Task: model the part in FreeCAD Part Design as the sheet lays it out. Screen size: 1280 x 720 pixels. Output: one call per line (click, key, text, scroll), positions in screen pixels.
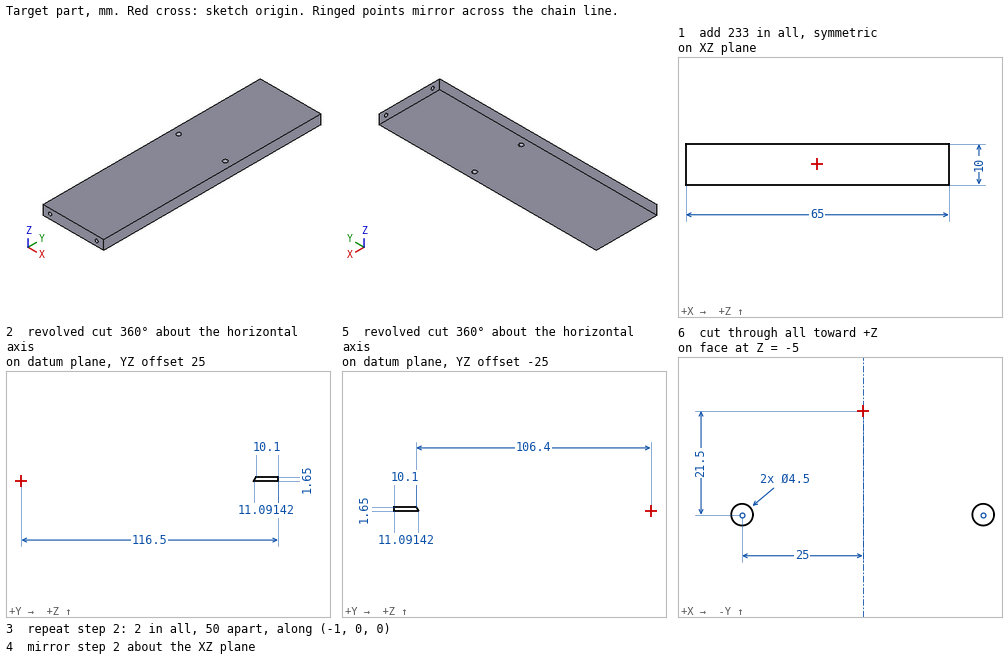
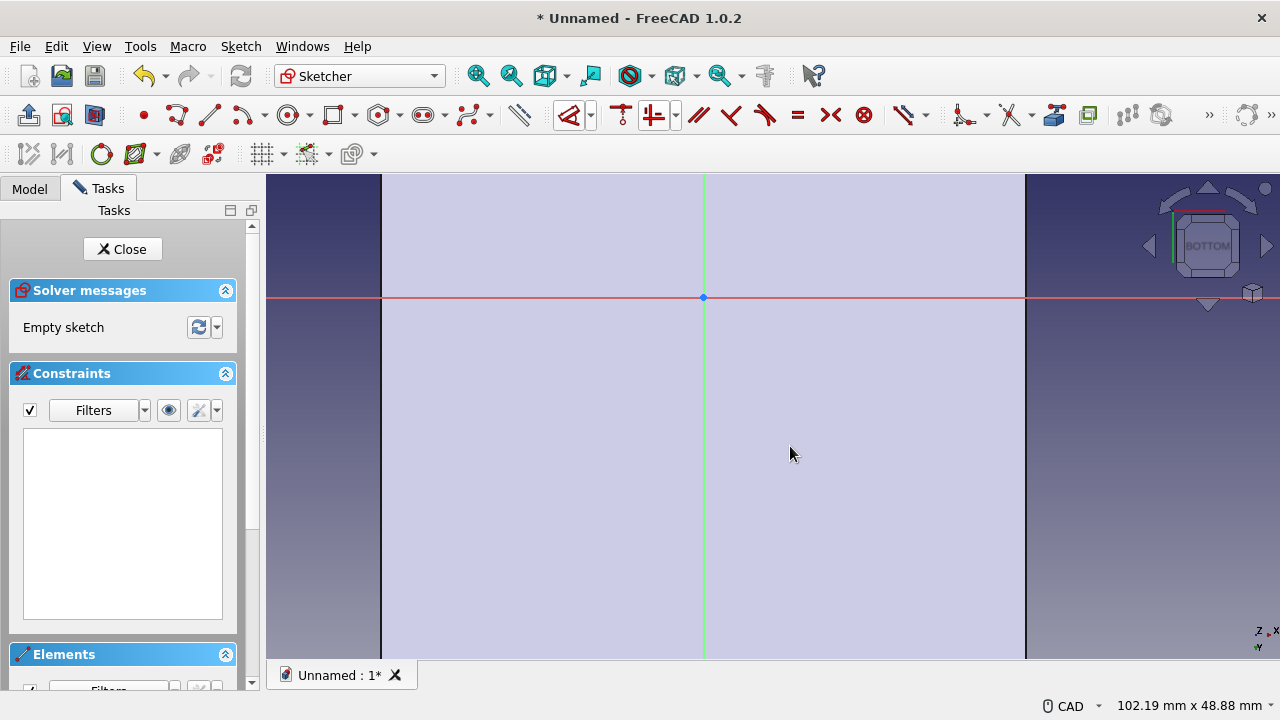
key(g)
key(c)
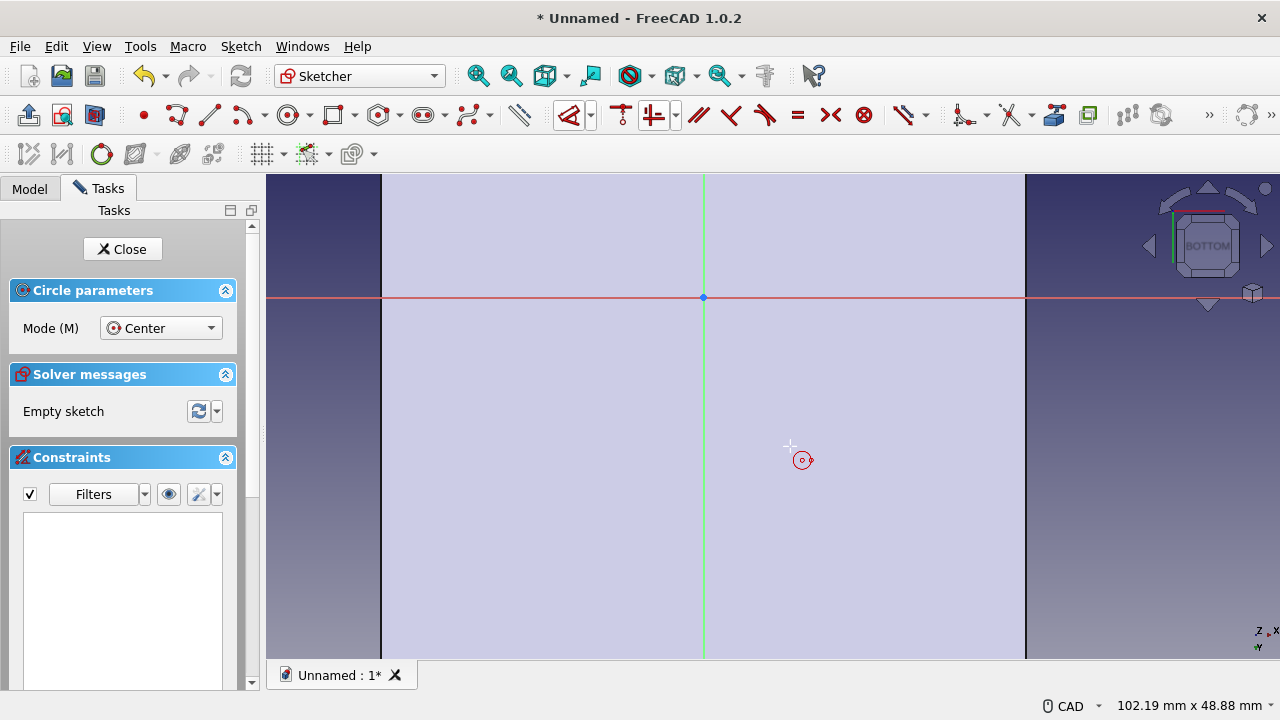
click(456, 511)
click(471, 495)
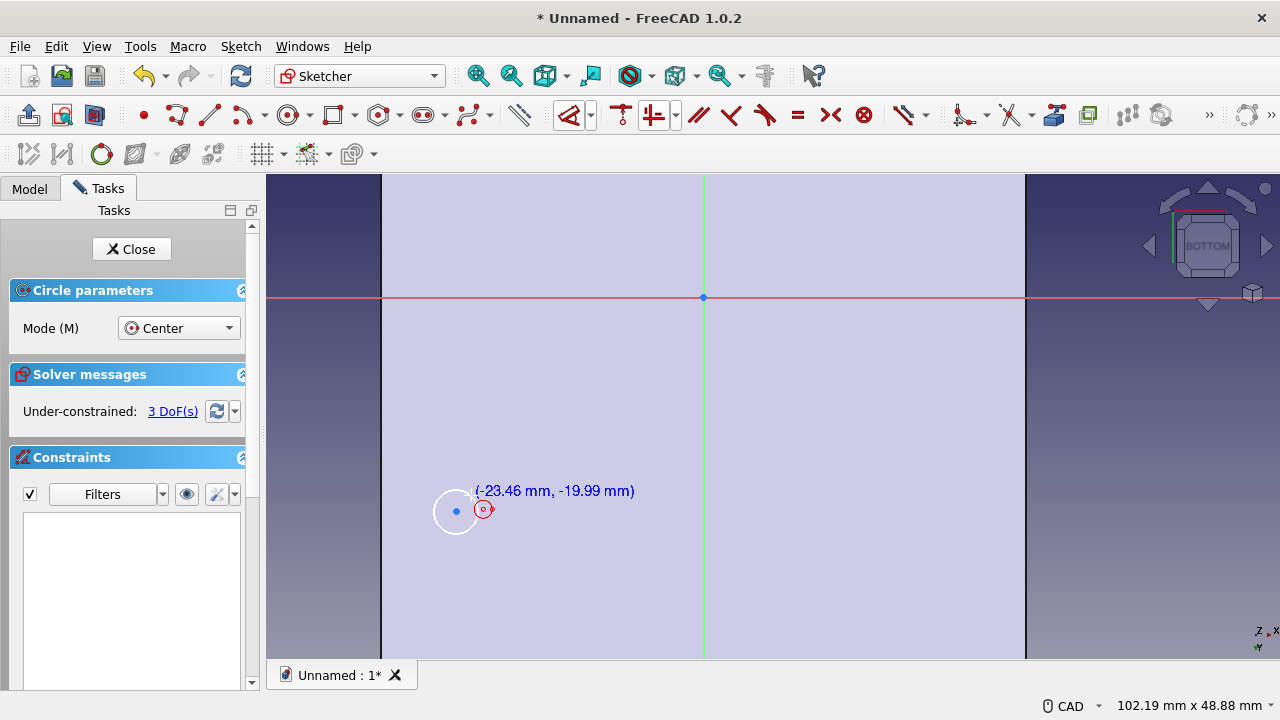
click(952, 511)
click(968, 495)
key(Escape)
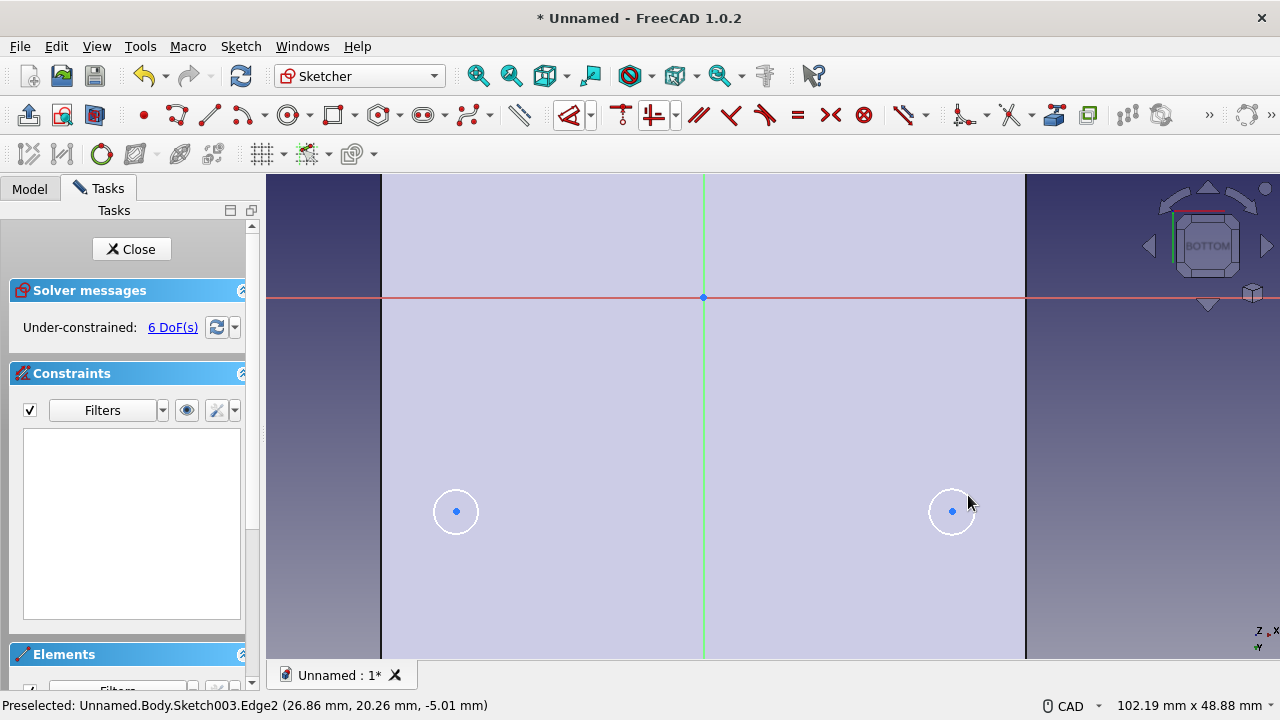
click(471, 496)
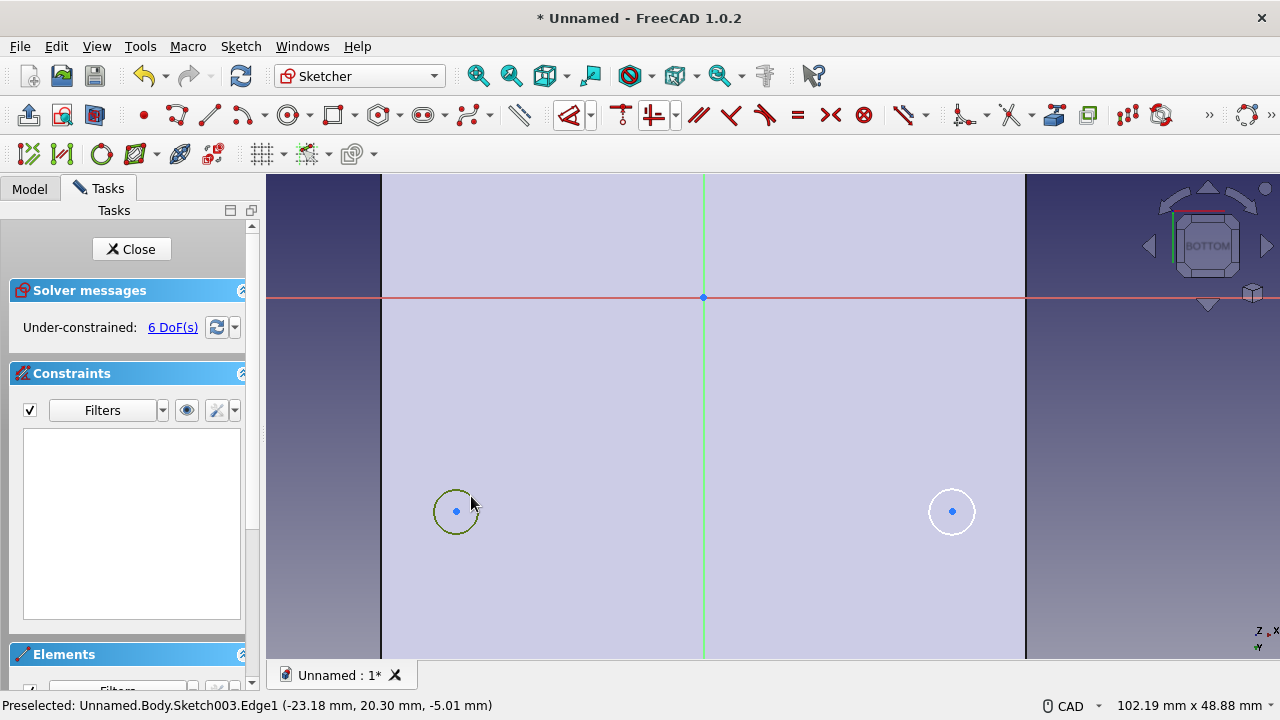
click(968, 496)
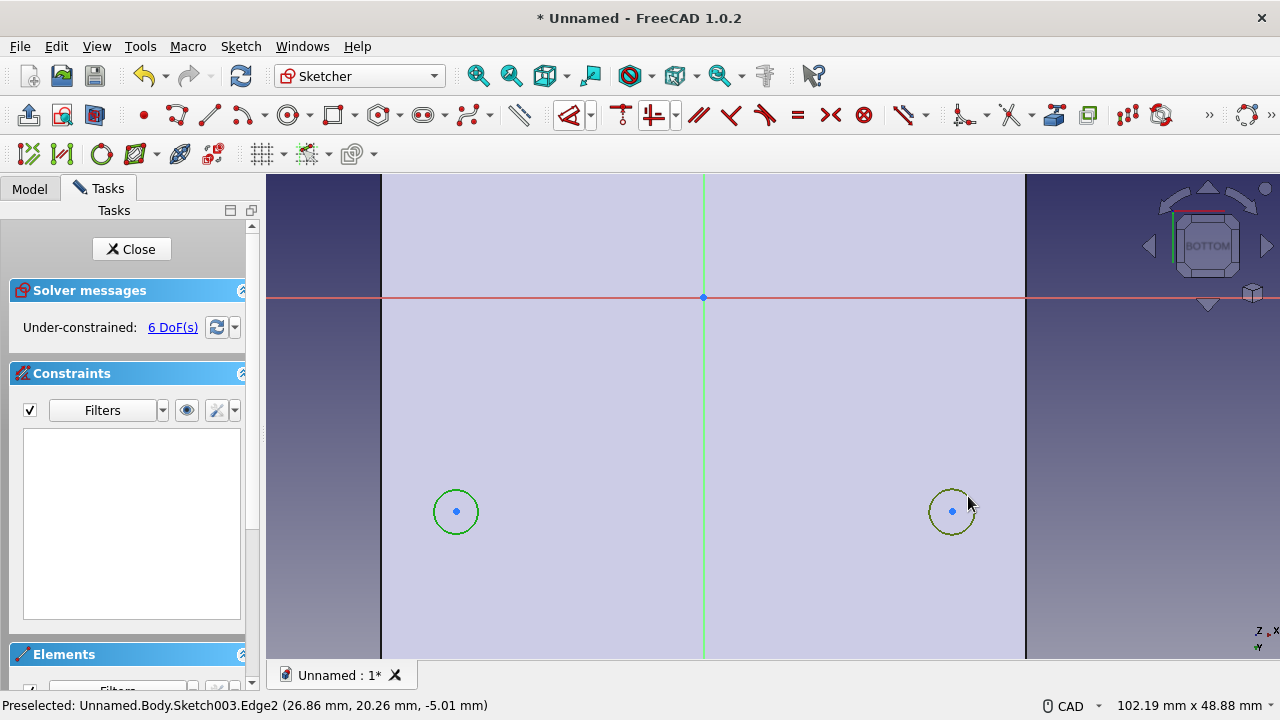
key(e)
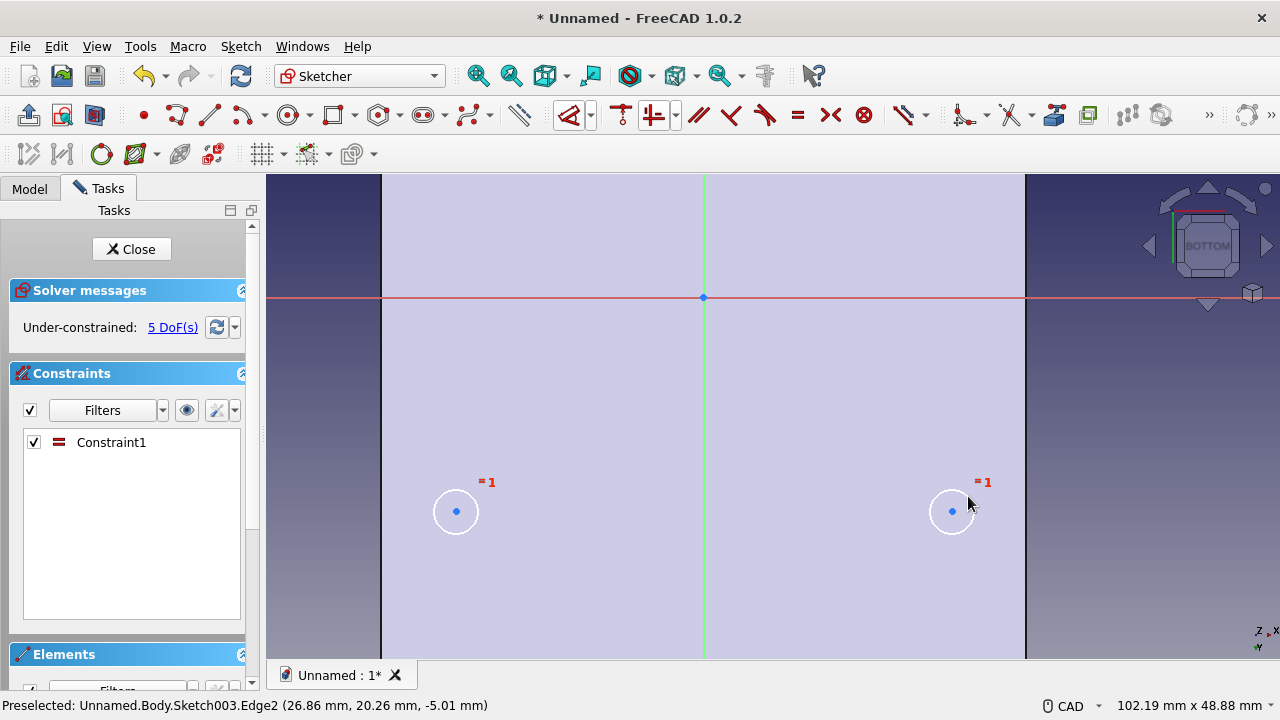
click(456, 512)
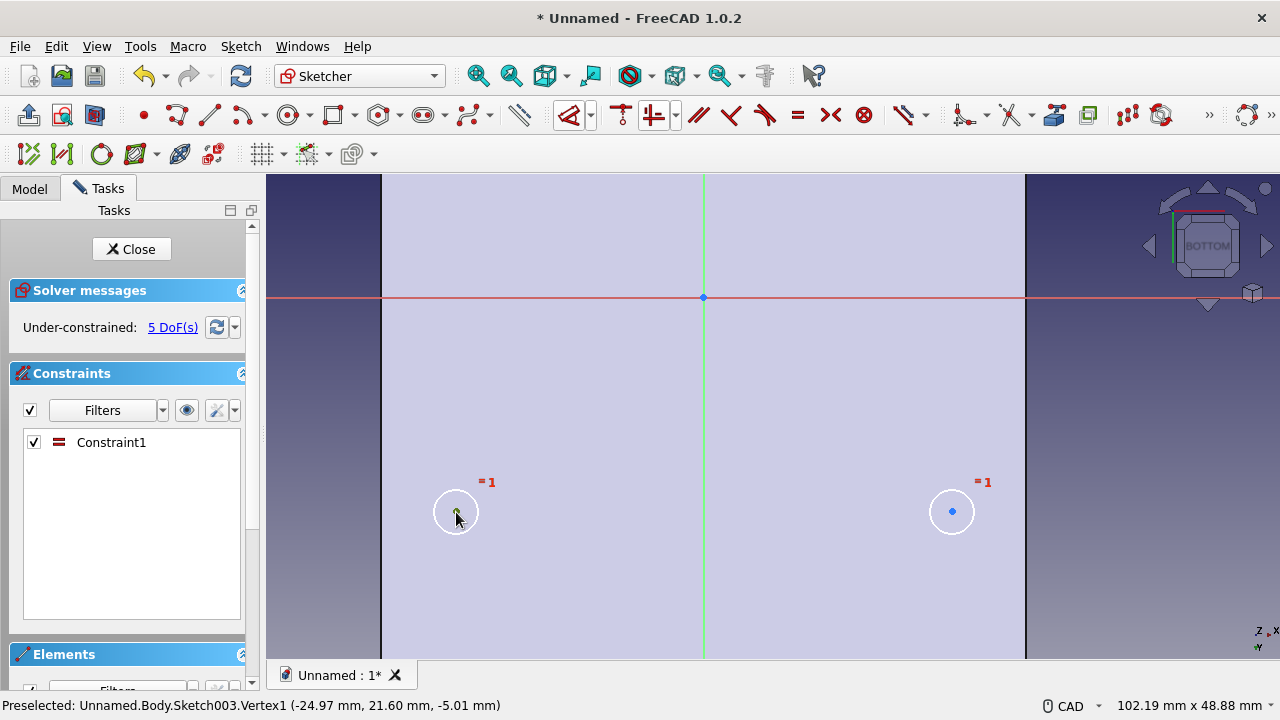
click(952, 512)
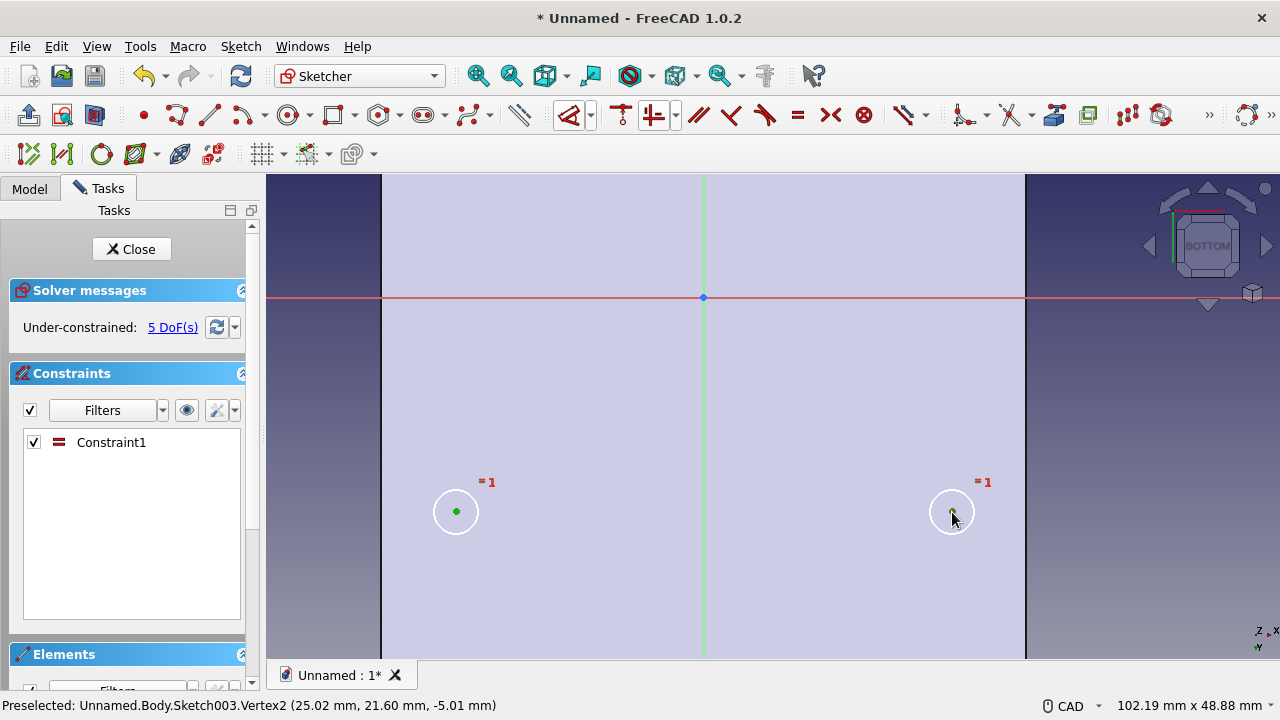
click(704, 600)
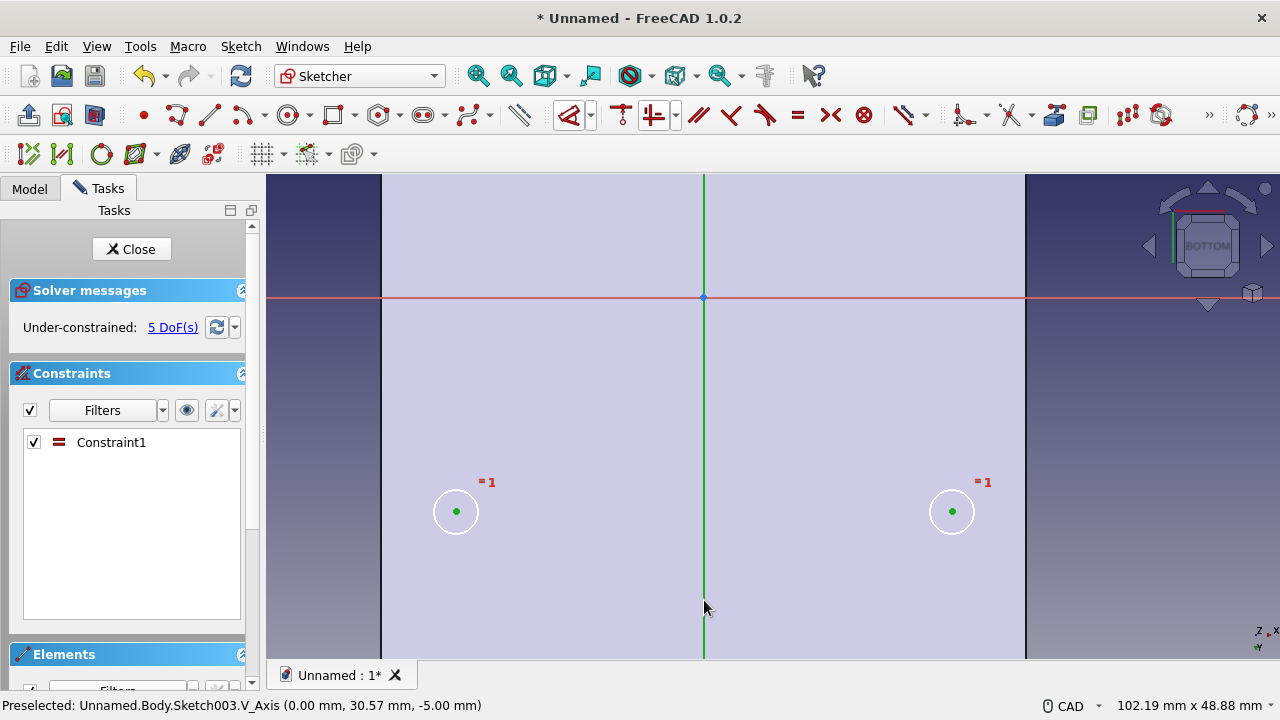
click(831, 116)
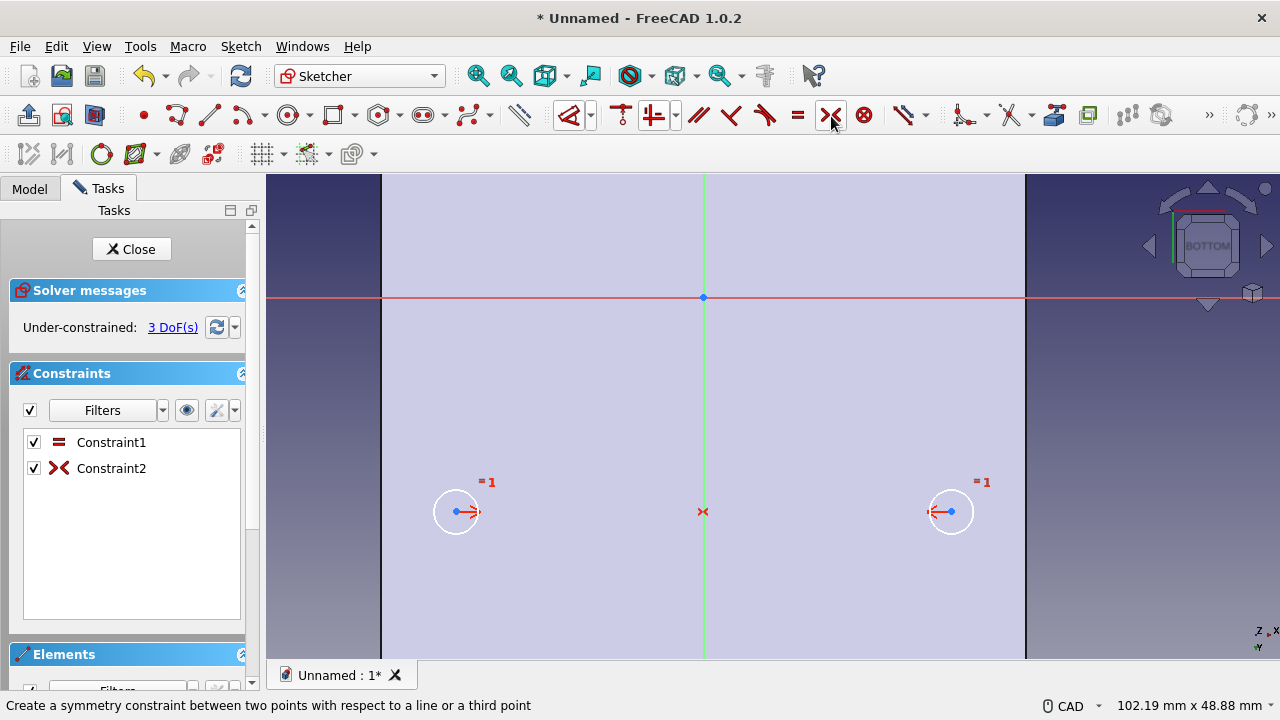
key(d)